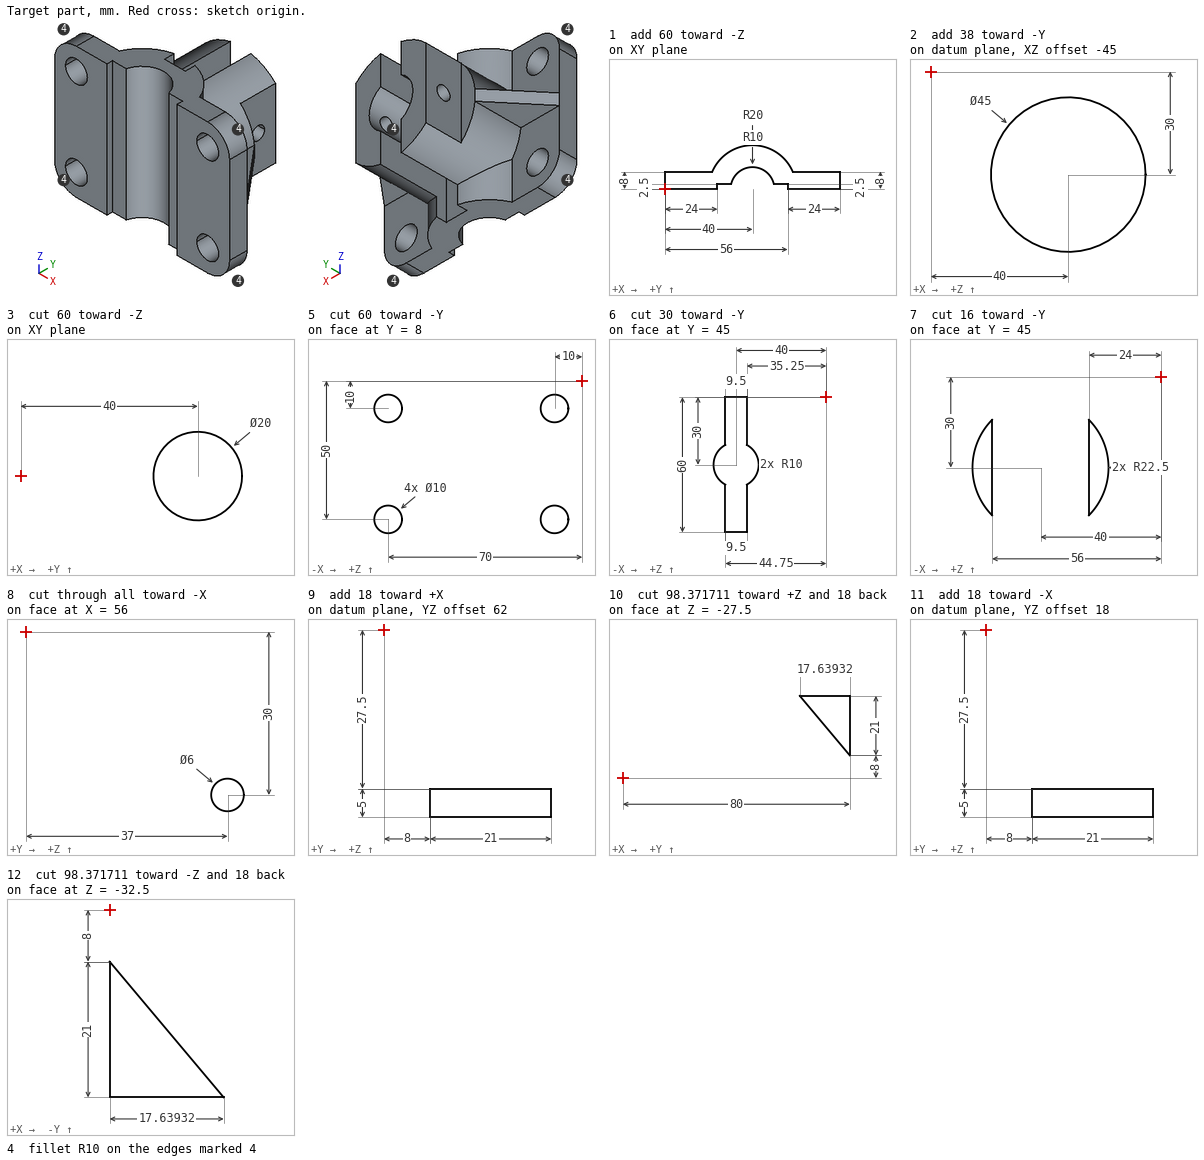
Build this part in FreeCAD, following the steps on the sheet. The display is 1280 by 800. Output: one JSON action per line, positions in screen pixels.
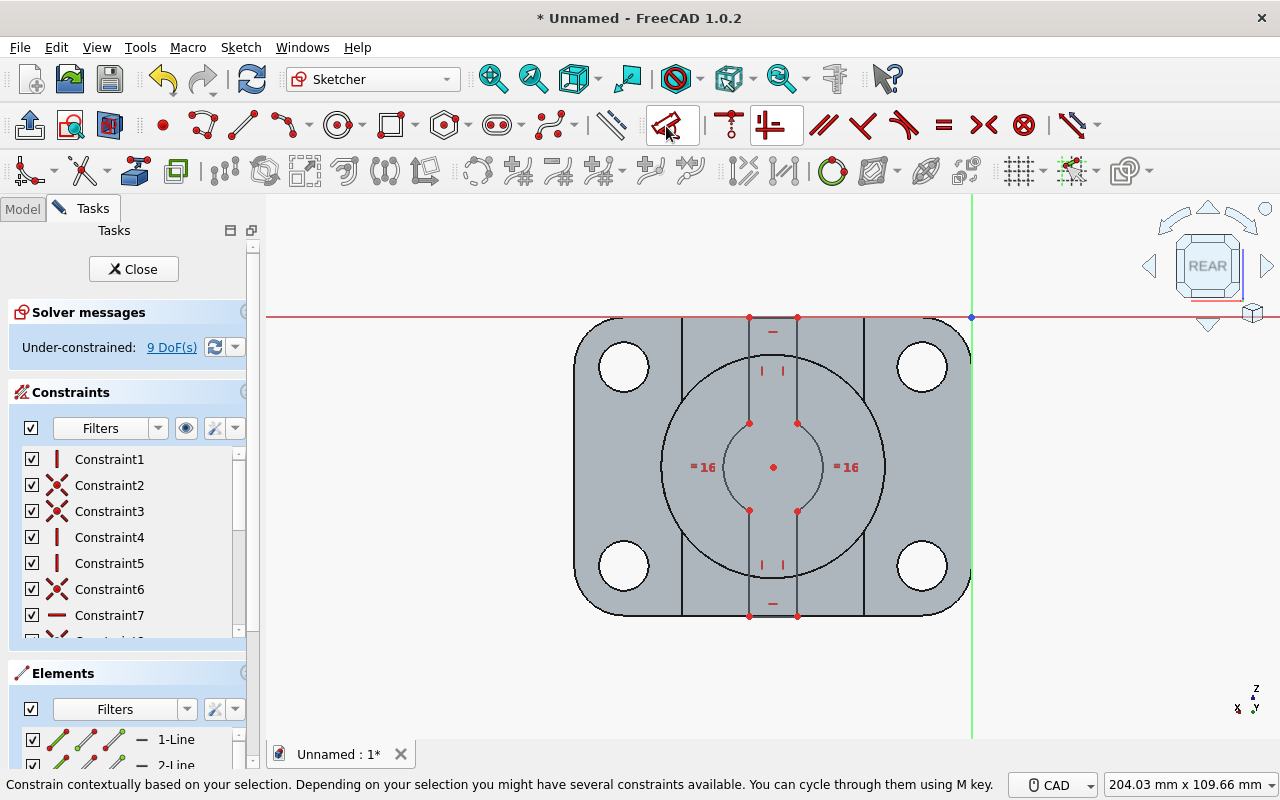
{"action": "left_click", "coordinate": [728, 447]}
{"action": "left_click", "coordinate": [699, 434]}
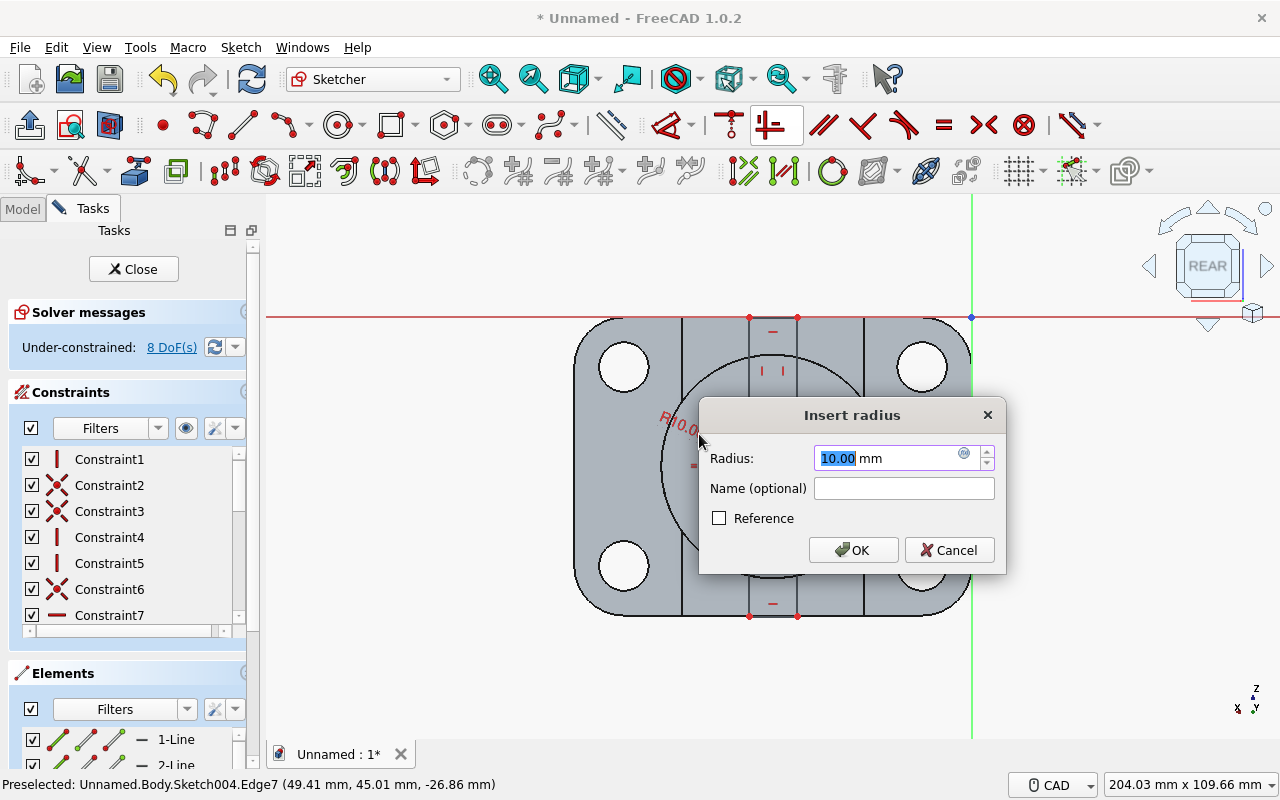
{"action": "type", "text": "10"}
{"action": "key", "text": "Return"}
{"action": "key", "text": "Escape"}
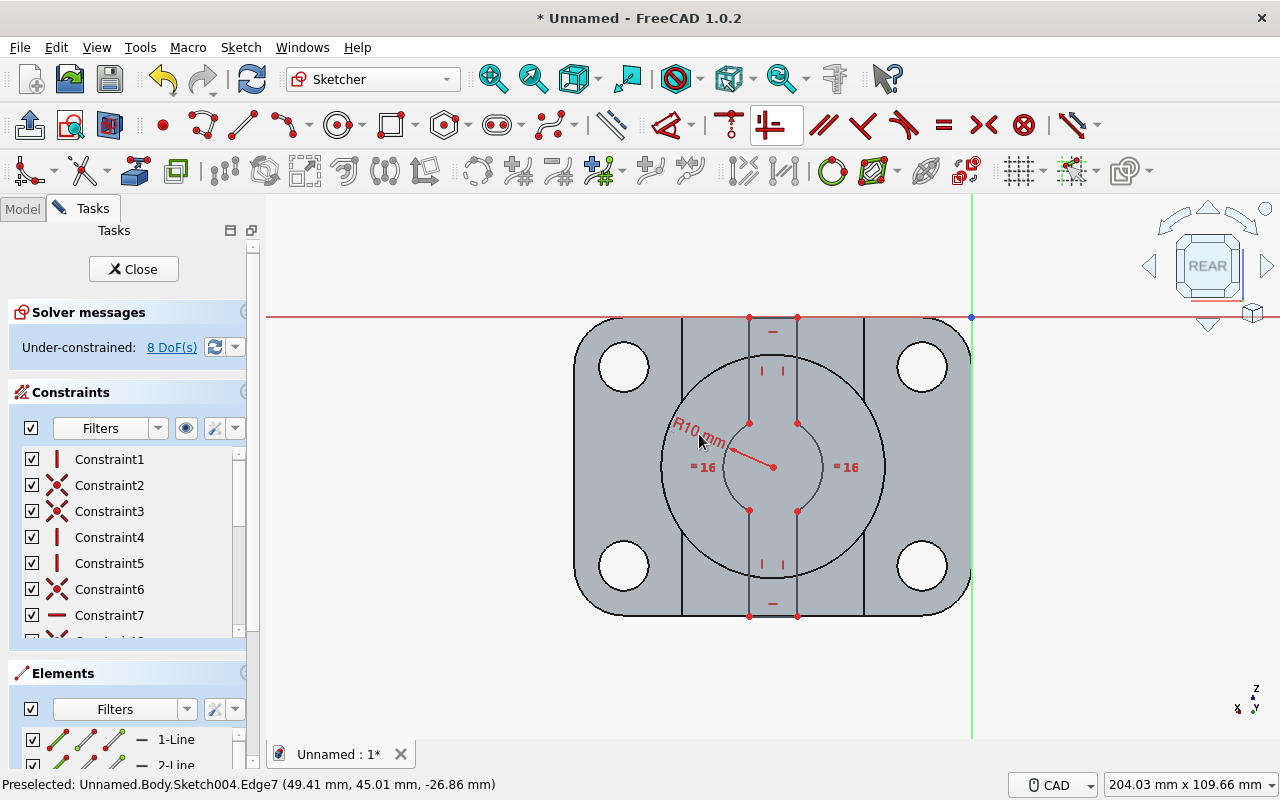
{"action": "left_click", "coordinate": [797, 318]}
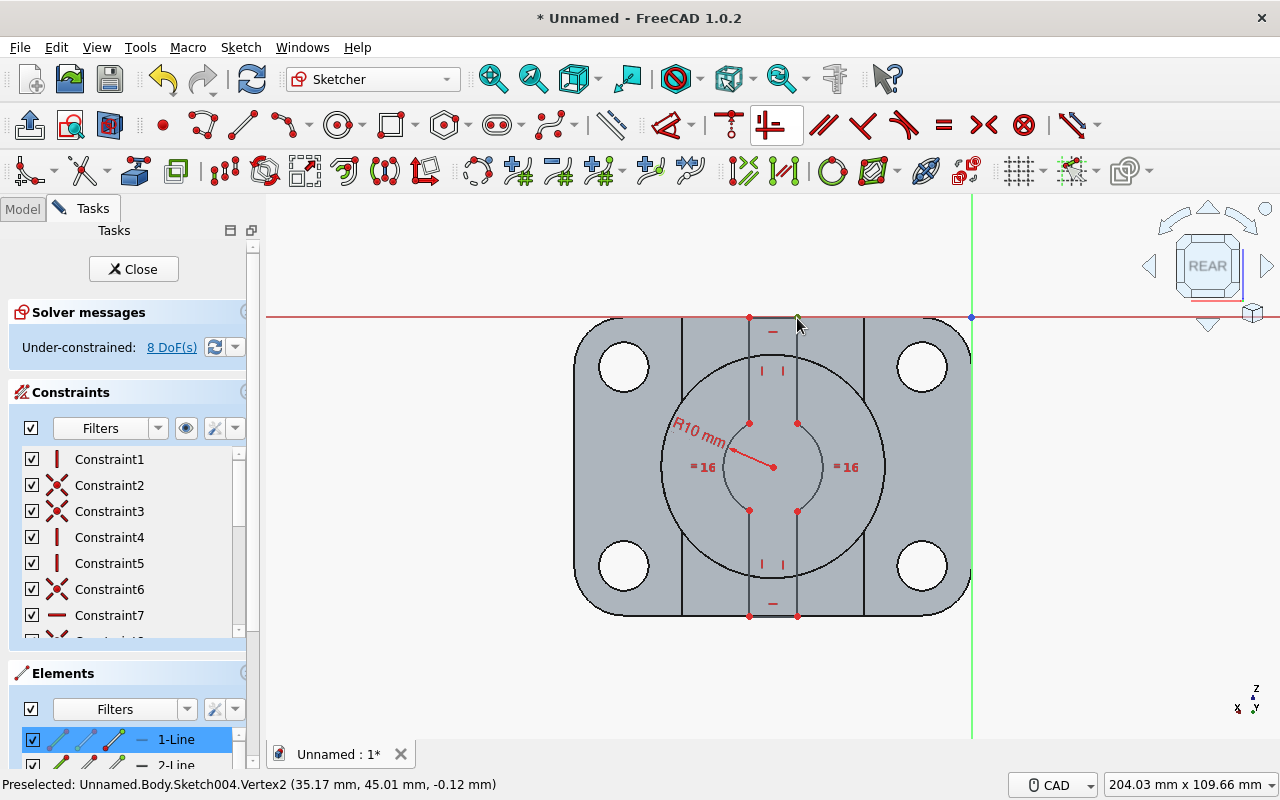
{"action": "left_click", "coordinate": [353, 317]}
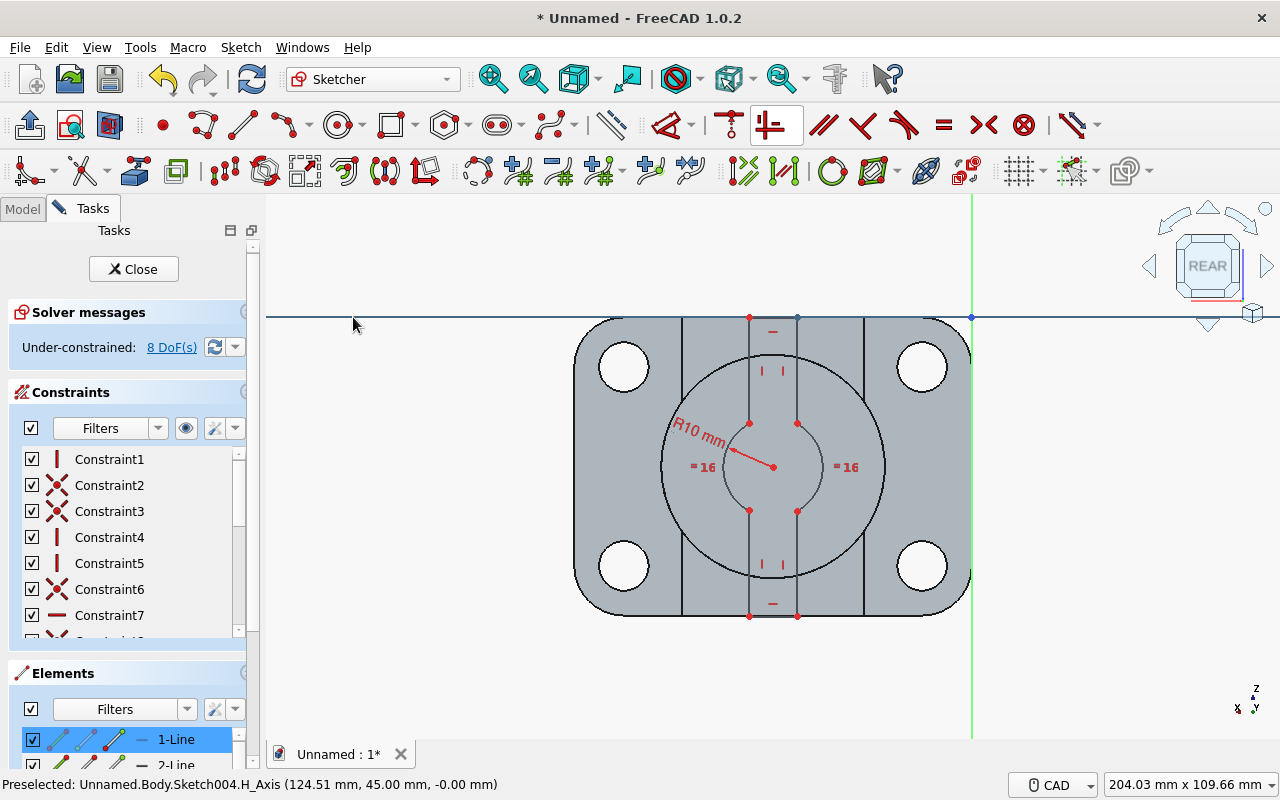
{"action": "left_click", "coordinate": [730, 126]}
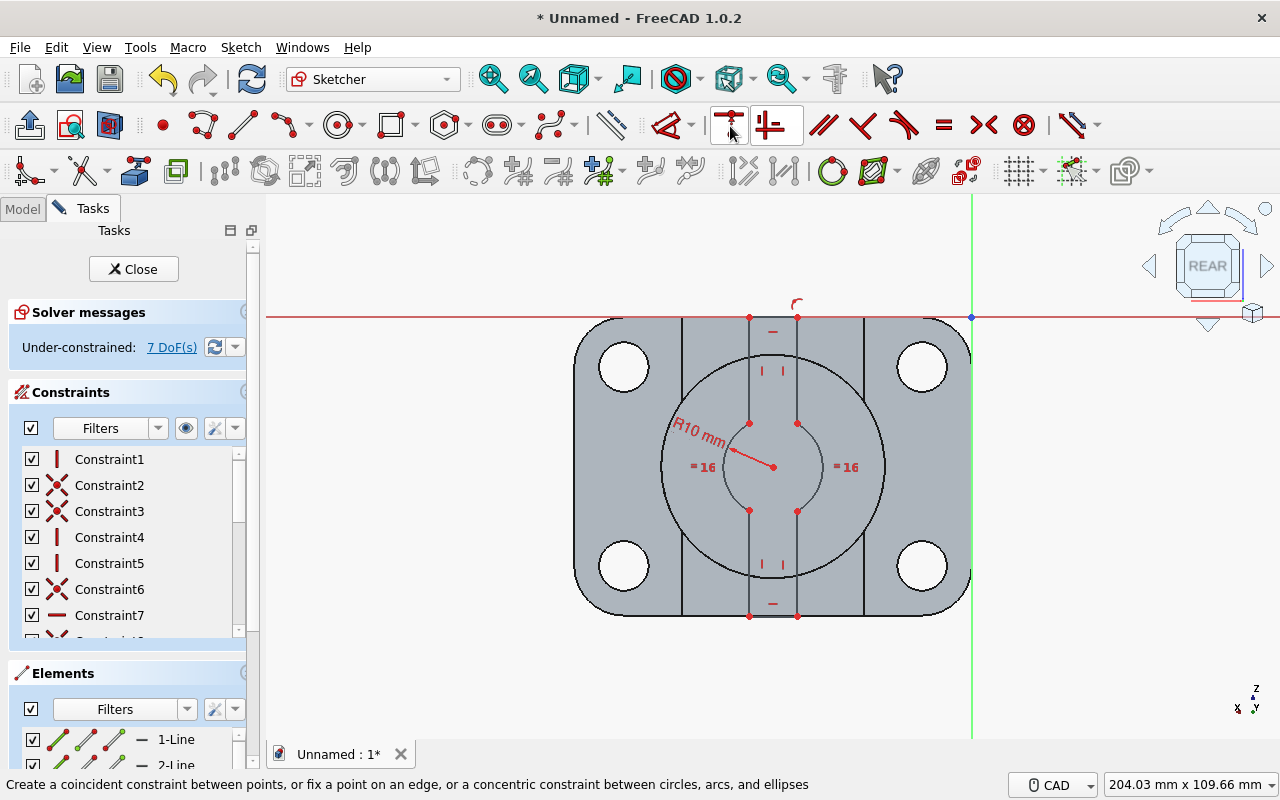
{"action": "left_click", "coordinate": [666, 126]}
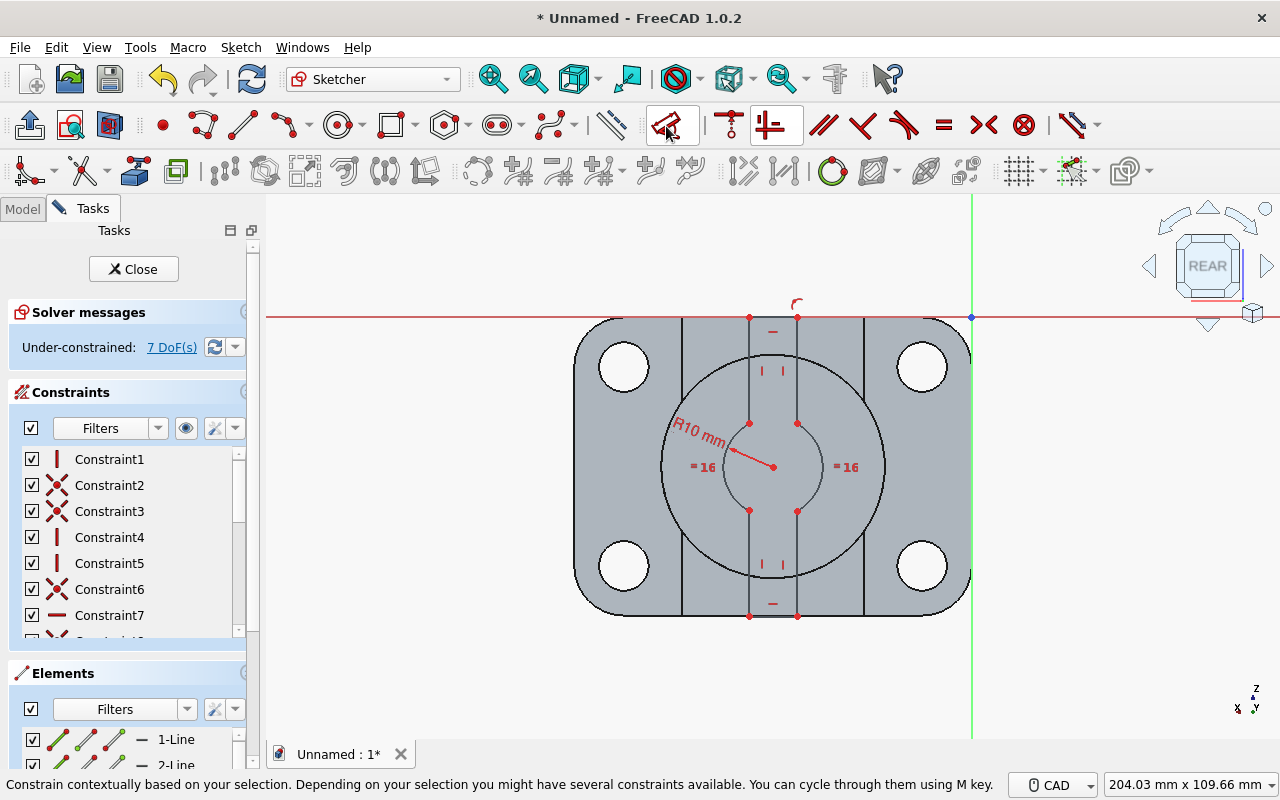
{"action": "left_click", "coordinate": [783, 317]}
{"action": "left_click", "coordinate": [773, 283]}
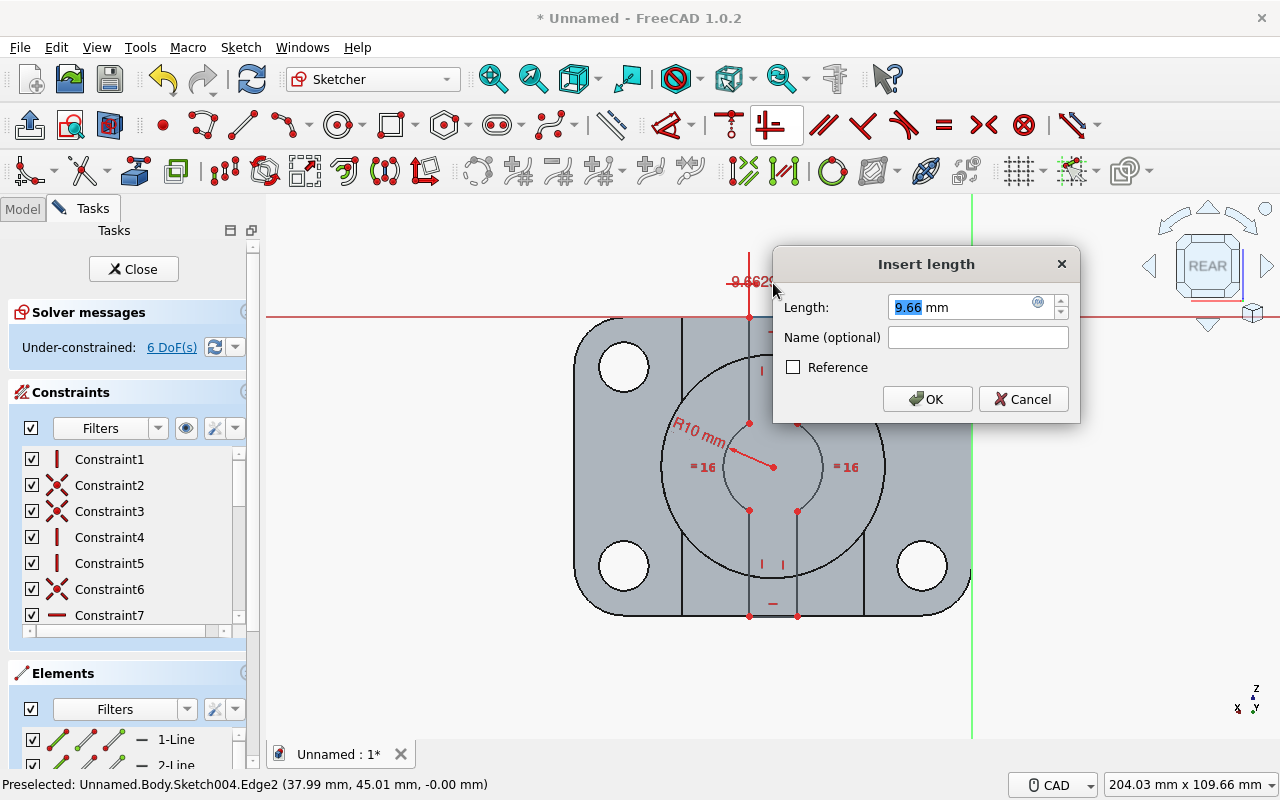
{"action": "type", "text": "9.5"}
{"action": "key", "text": "Return"}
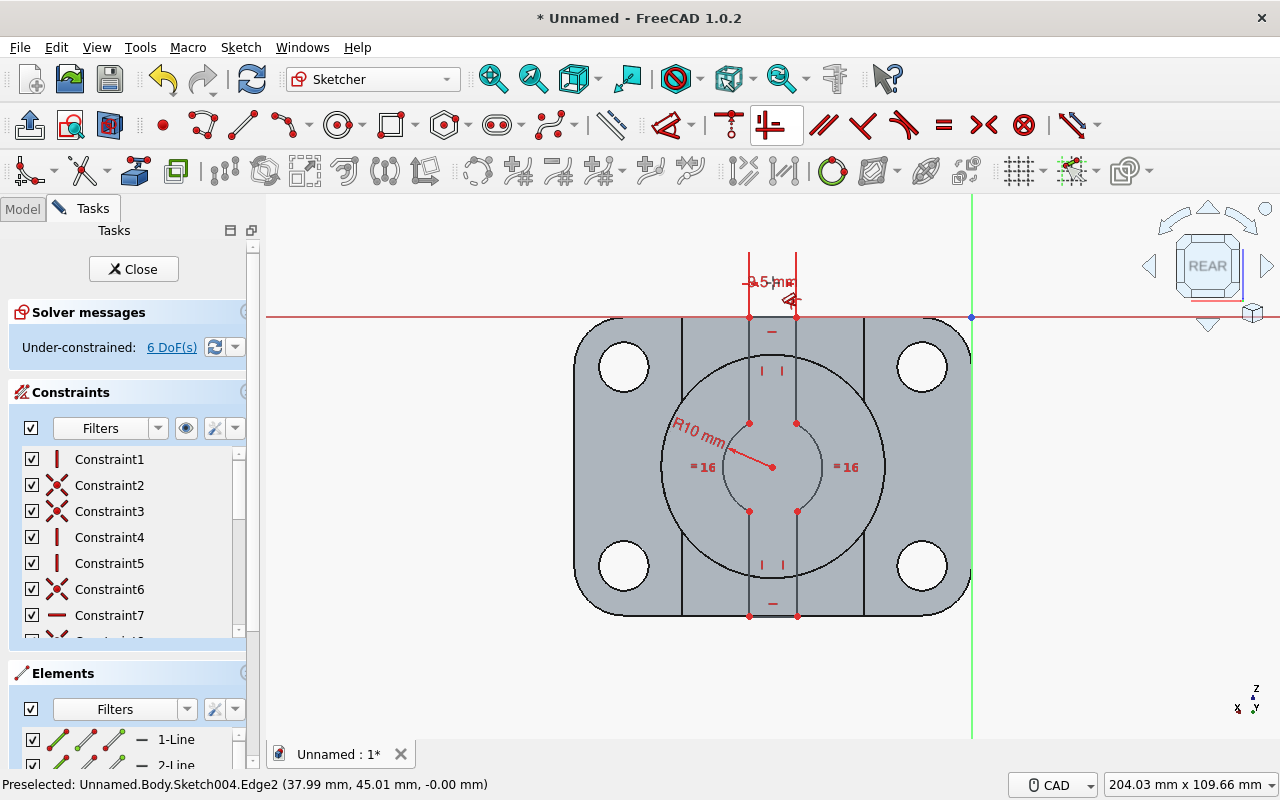
{"action": "left_click", "coordinate": [763, 617]}
{"action": "left_click", "coordinate": [773, 651]}